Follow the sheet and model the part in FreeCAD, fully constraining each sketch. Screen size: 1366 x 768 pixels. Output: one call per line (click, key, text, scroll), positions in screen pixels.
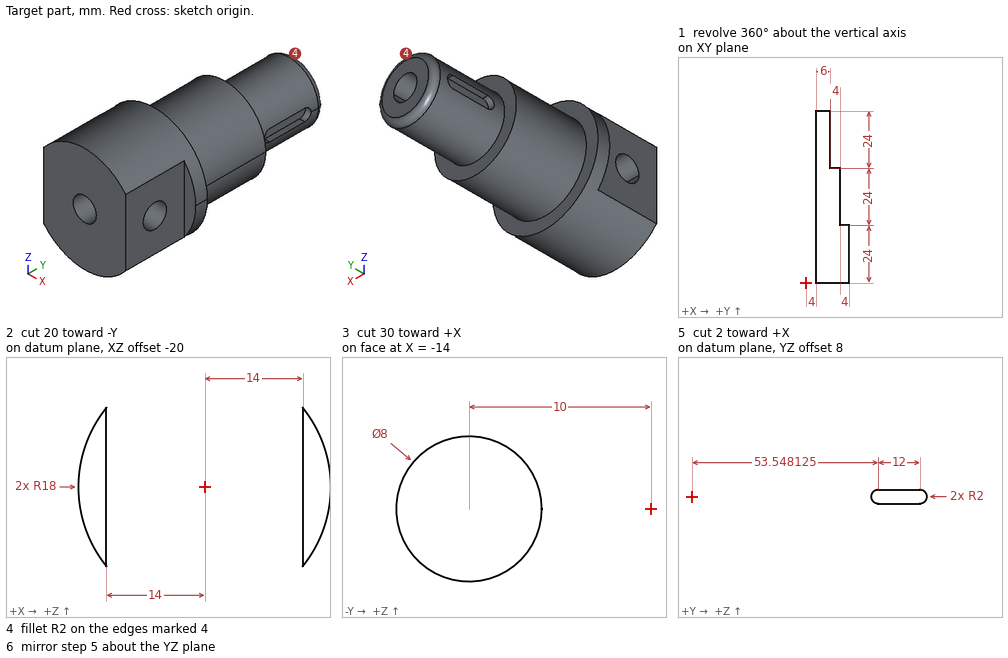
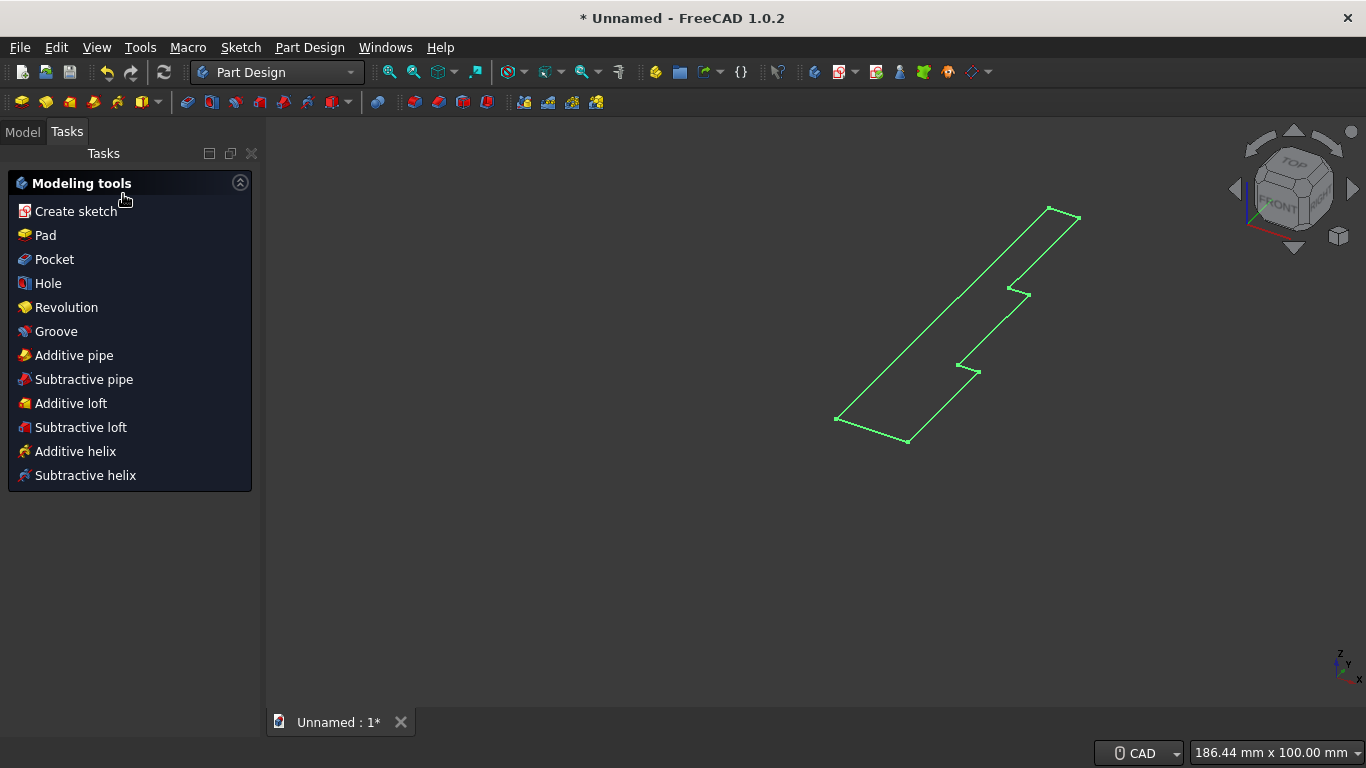
click(46, 102)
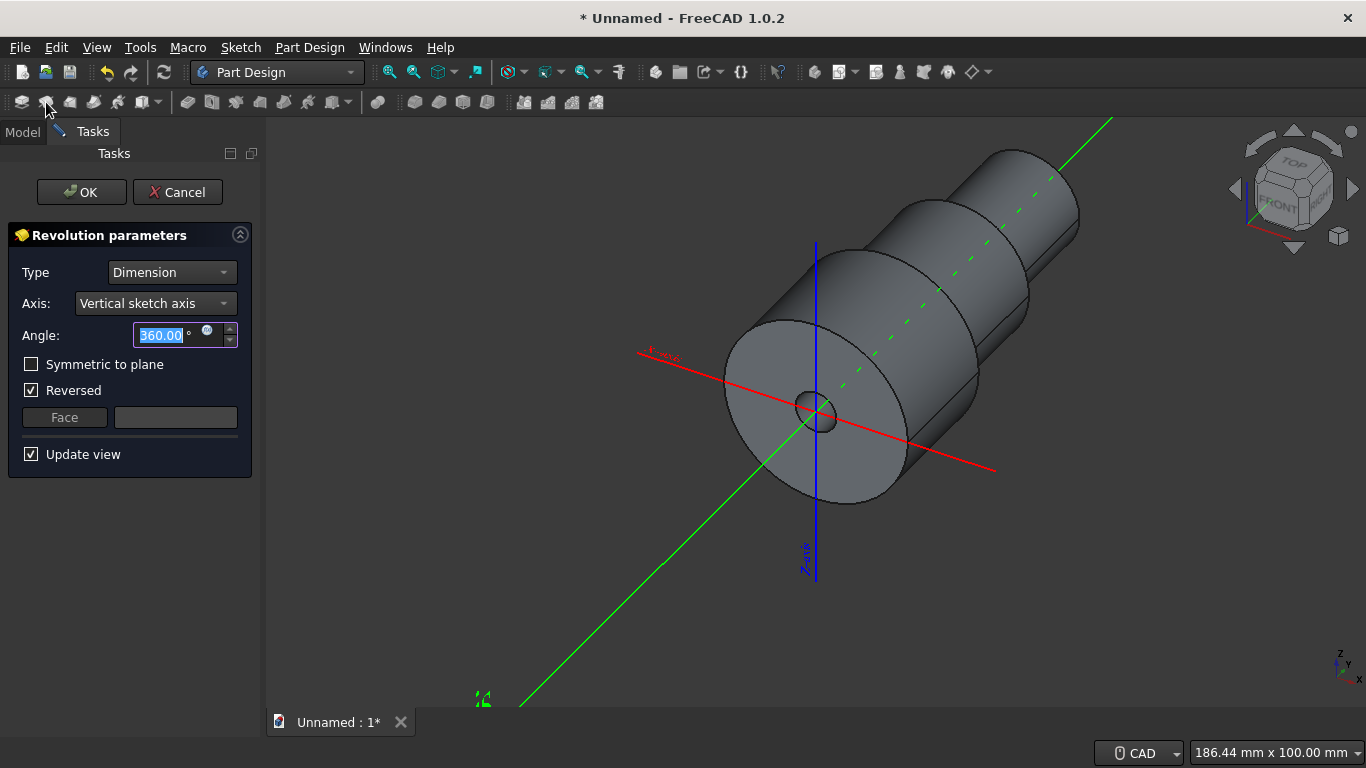
click(82, 192)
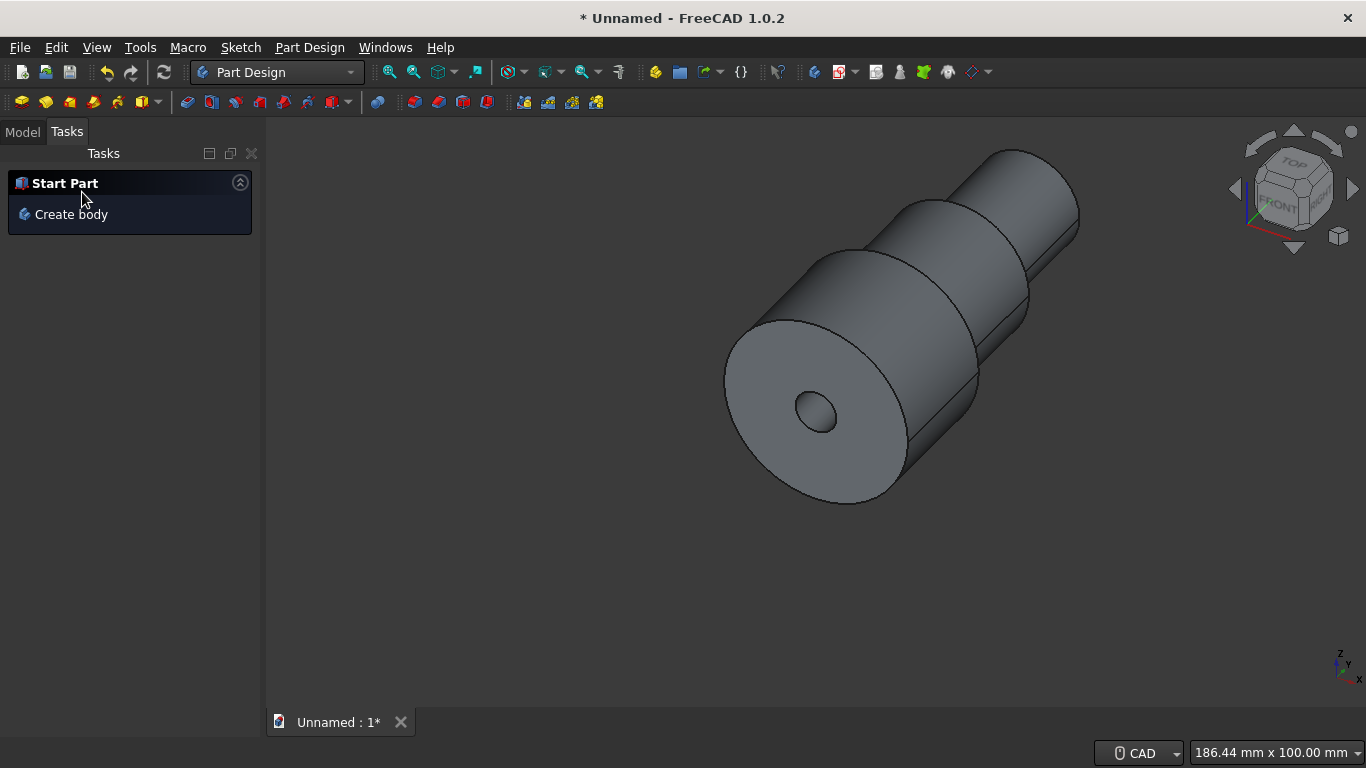
click(390, 72)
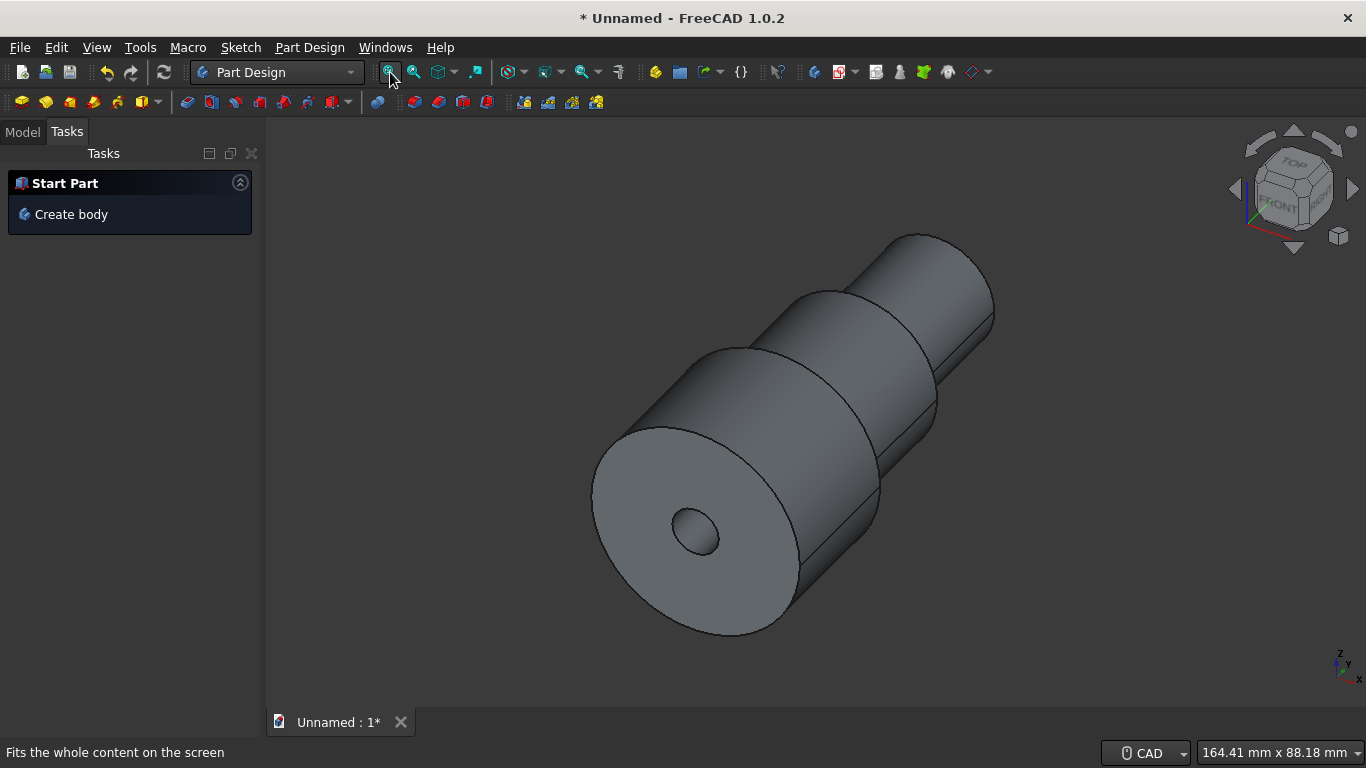
click(23, 131)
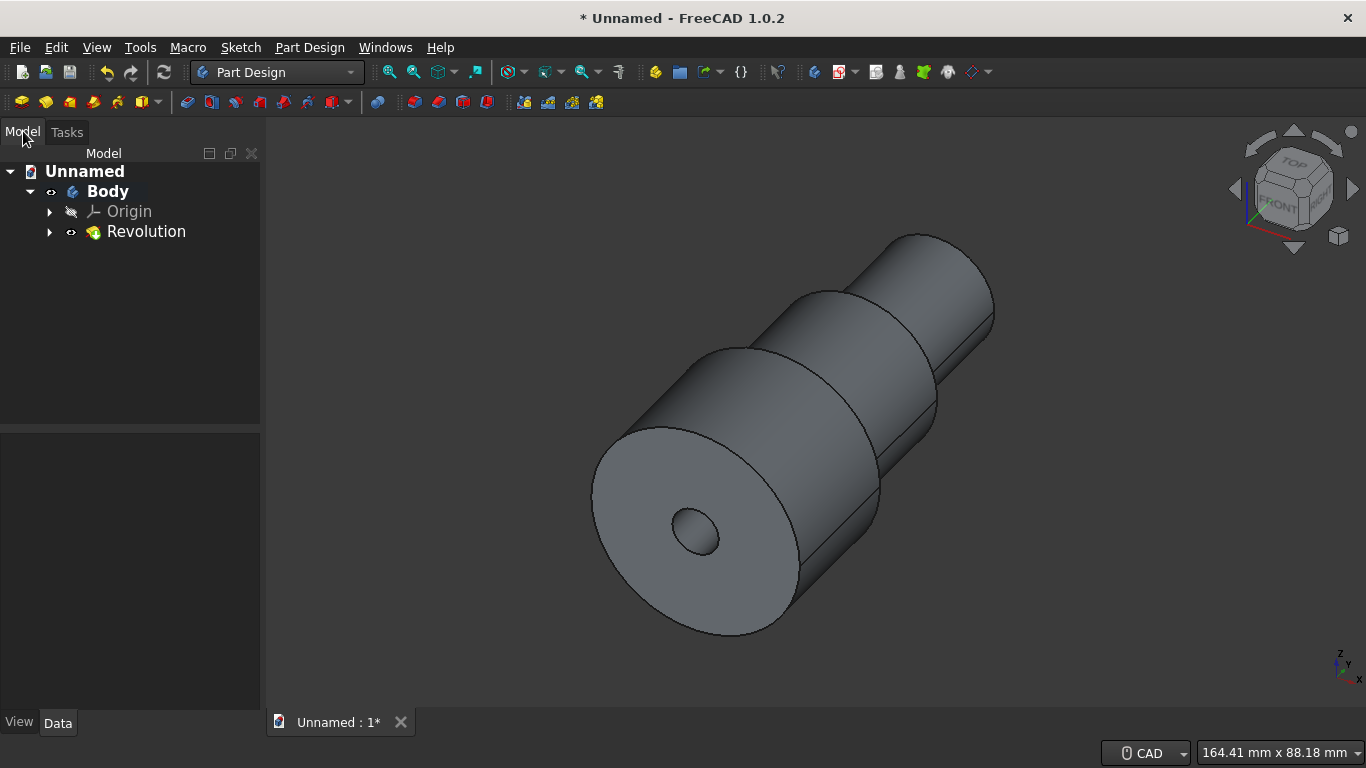
click(50, 212)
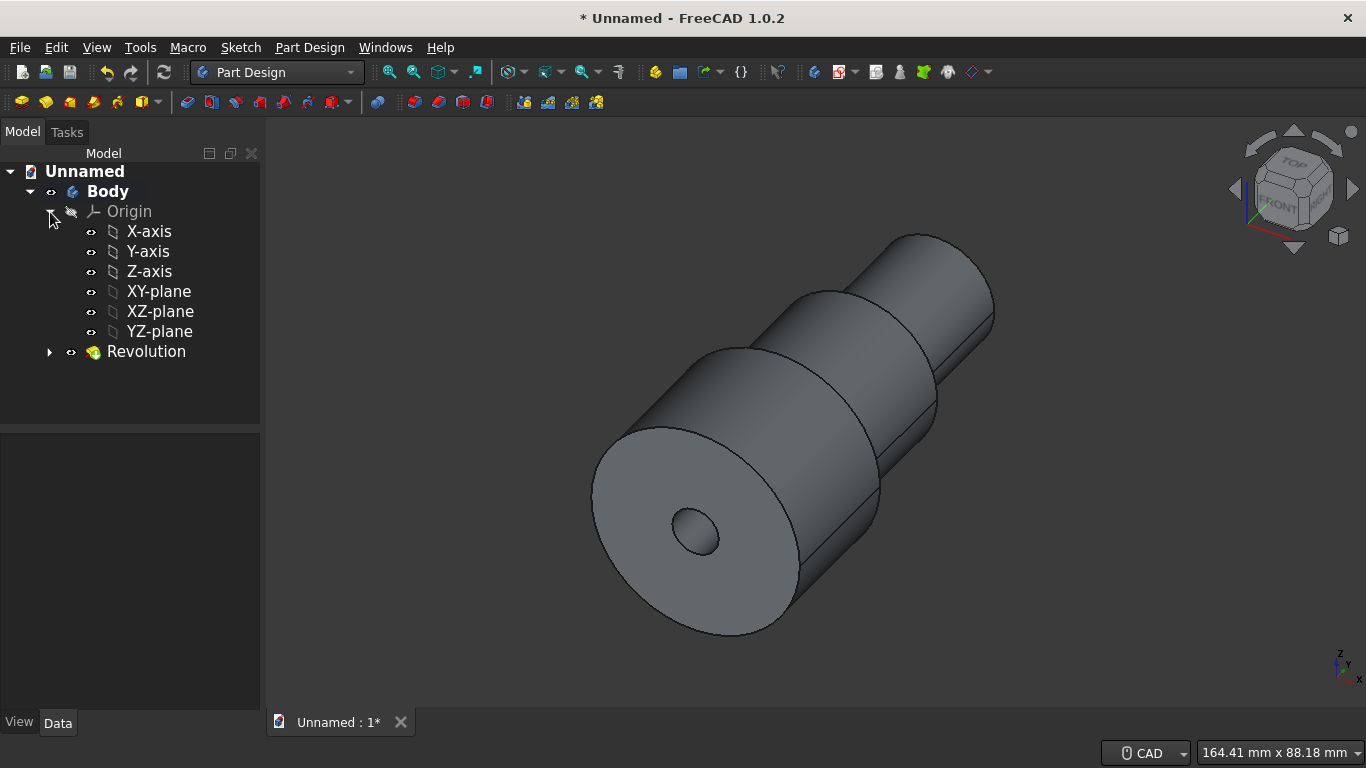
click(136, 312)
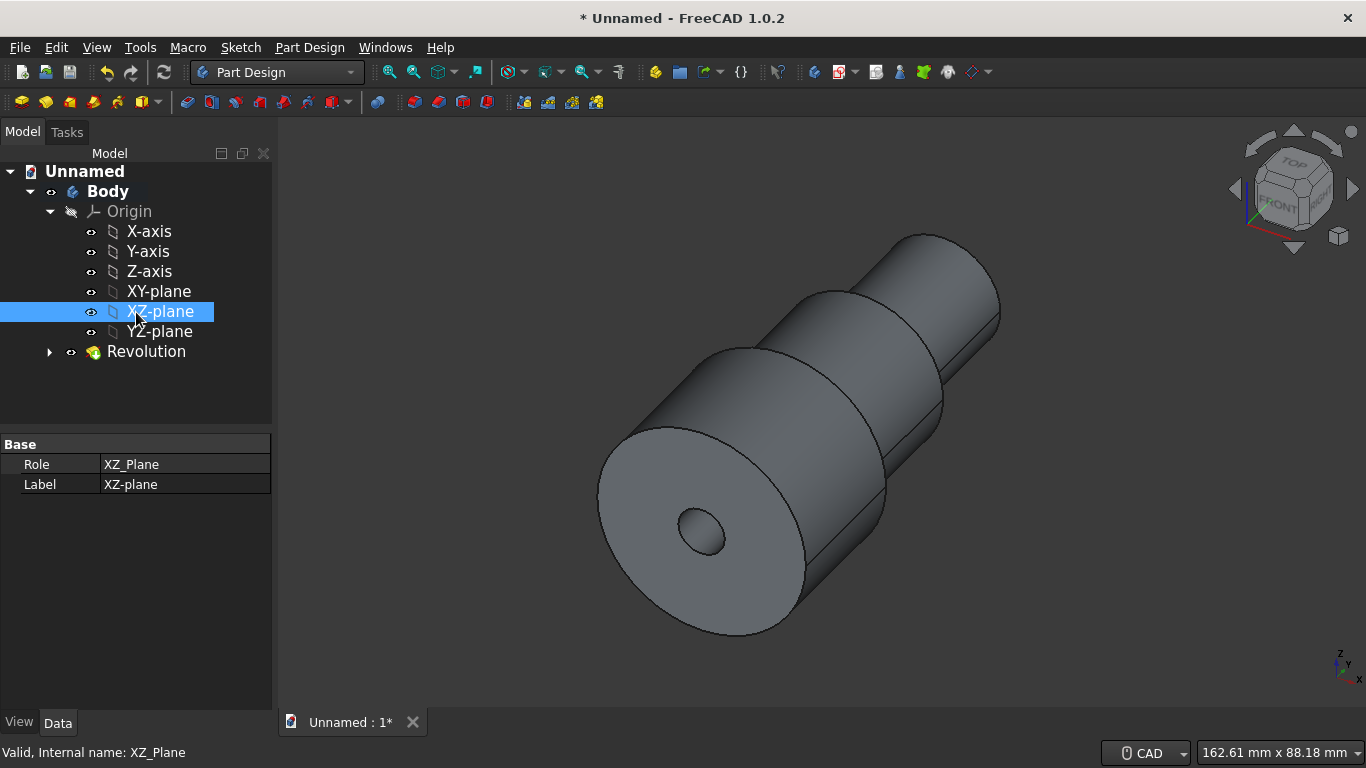
click(972, 72)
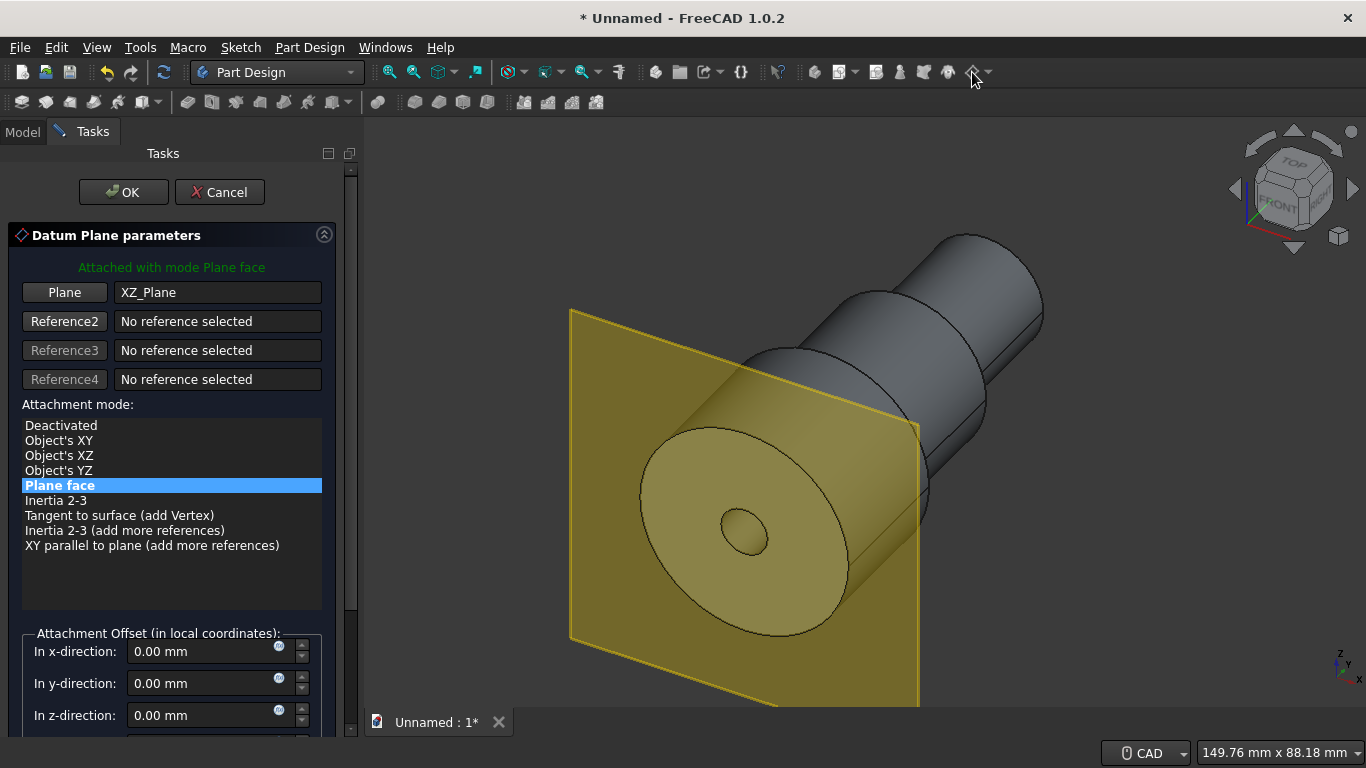
triple_click(210, 715)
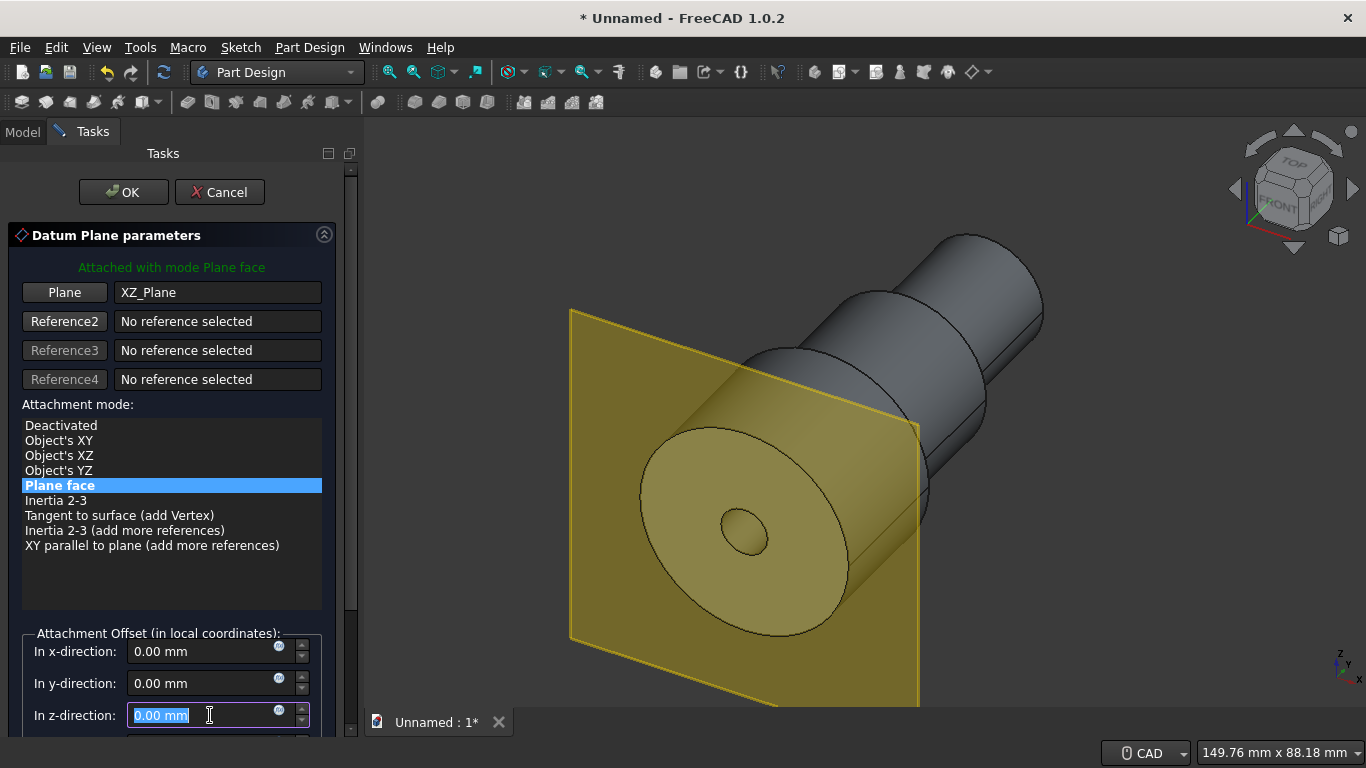
text(-20)
key(Tab)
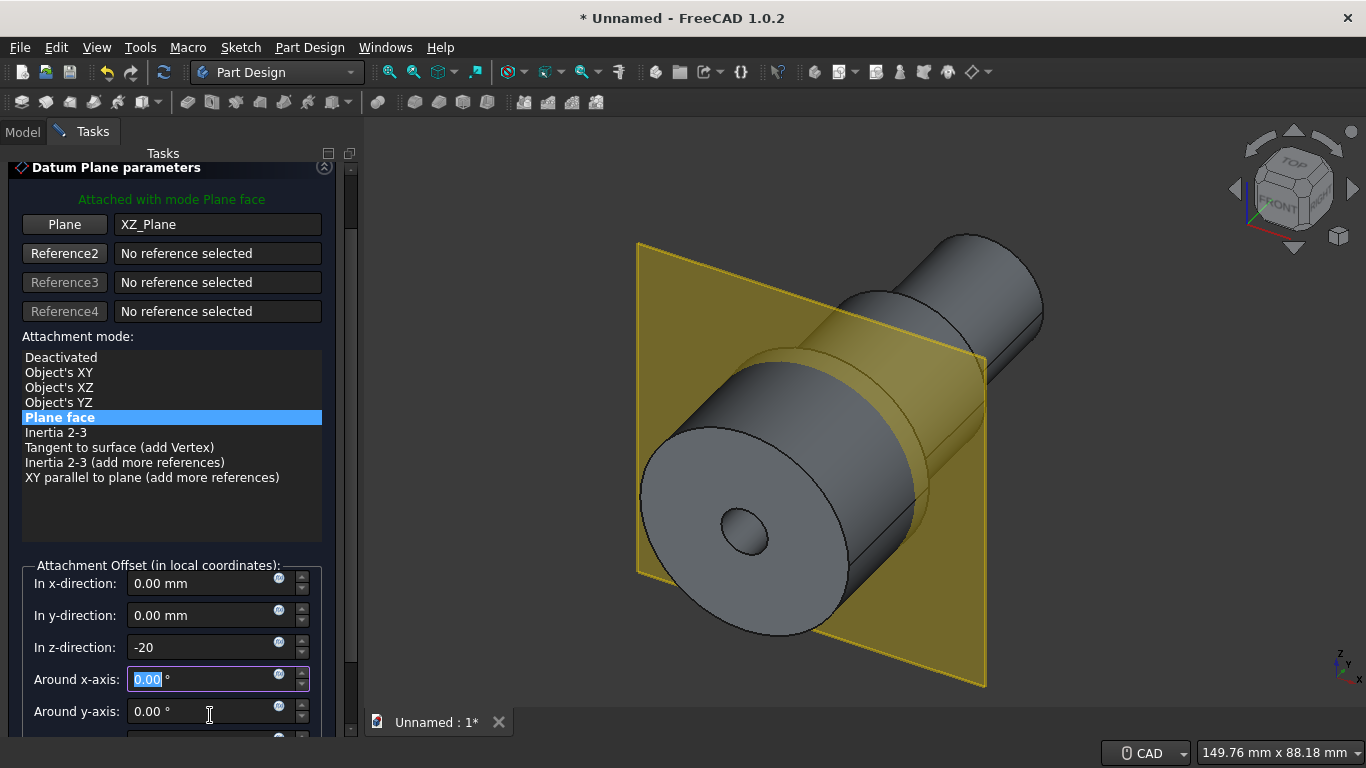
scroll(351, 450, up, 2)